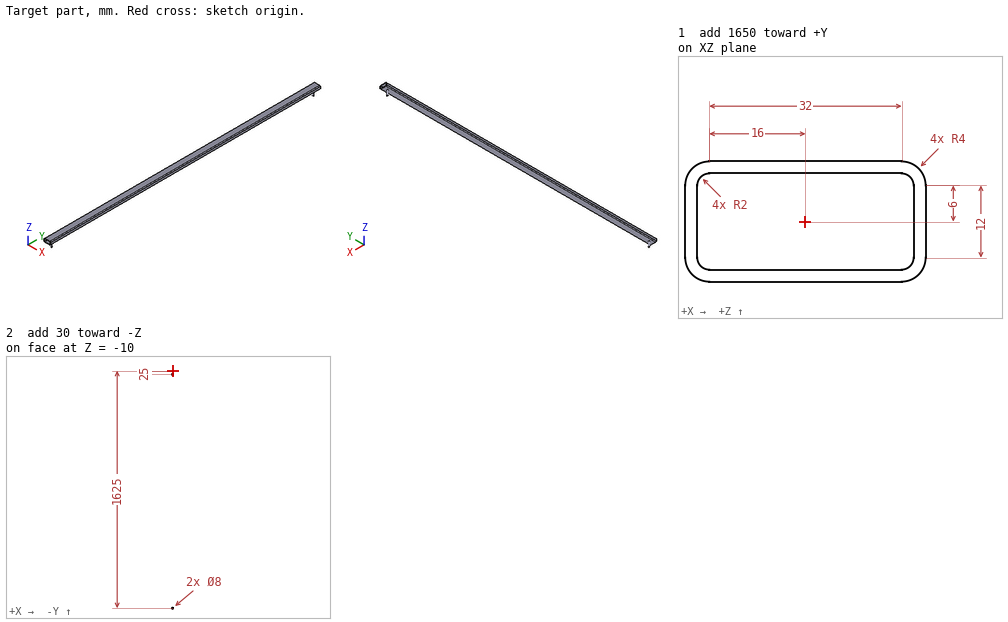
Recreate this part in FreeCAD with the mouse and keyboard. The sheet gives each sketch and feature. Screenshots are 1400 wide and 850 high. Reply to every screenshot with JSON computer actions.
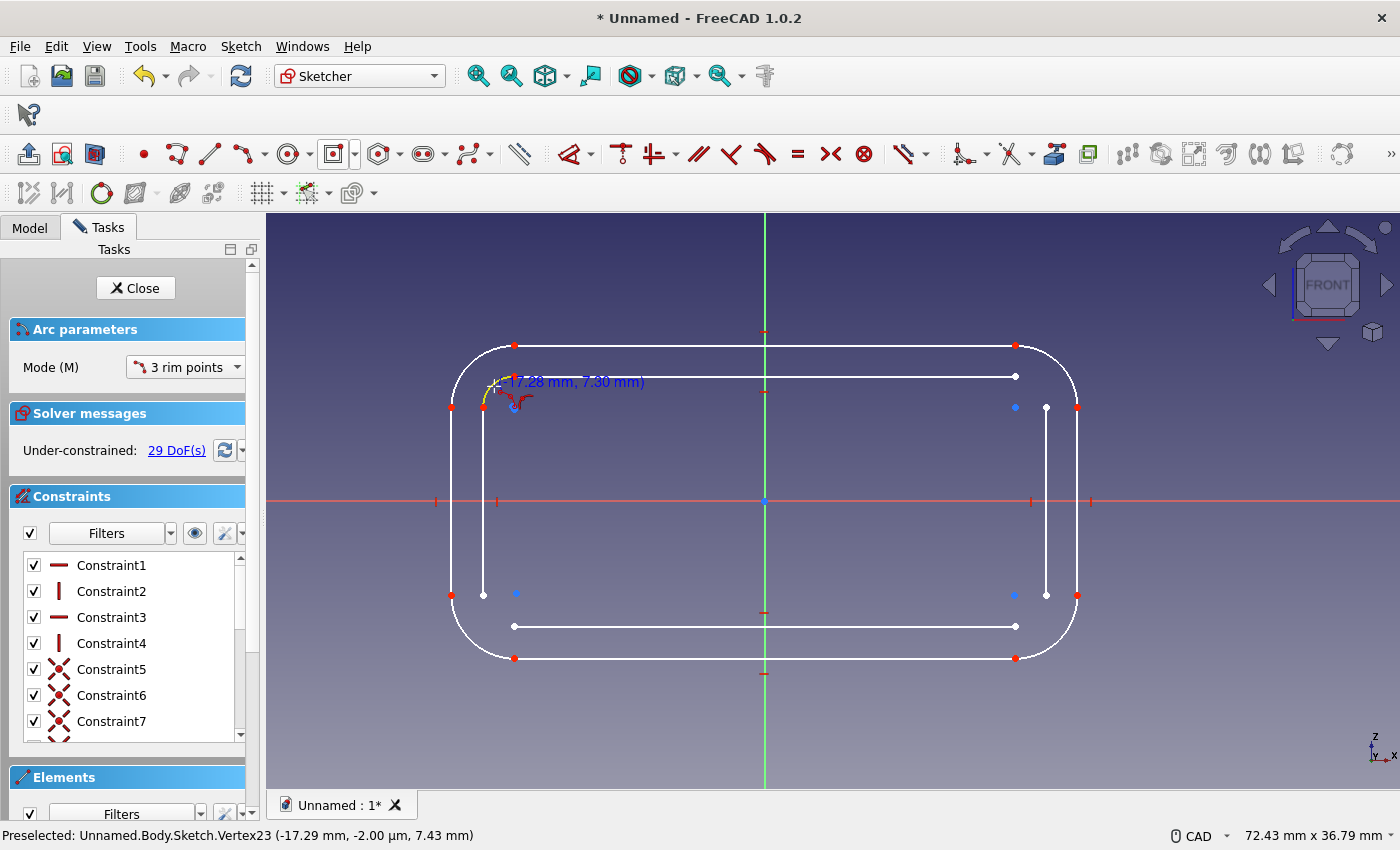
{"action": "left_click", "coordinate": [483, 596]}
{"action": "left_click", "coordinate": [514, 627]}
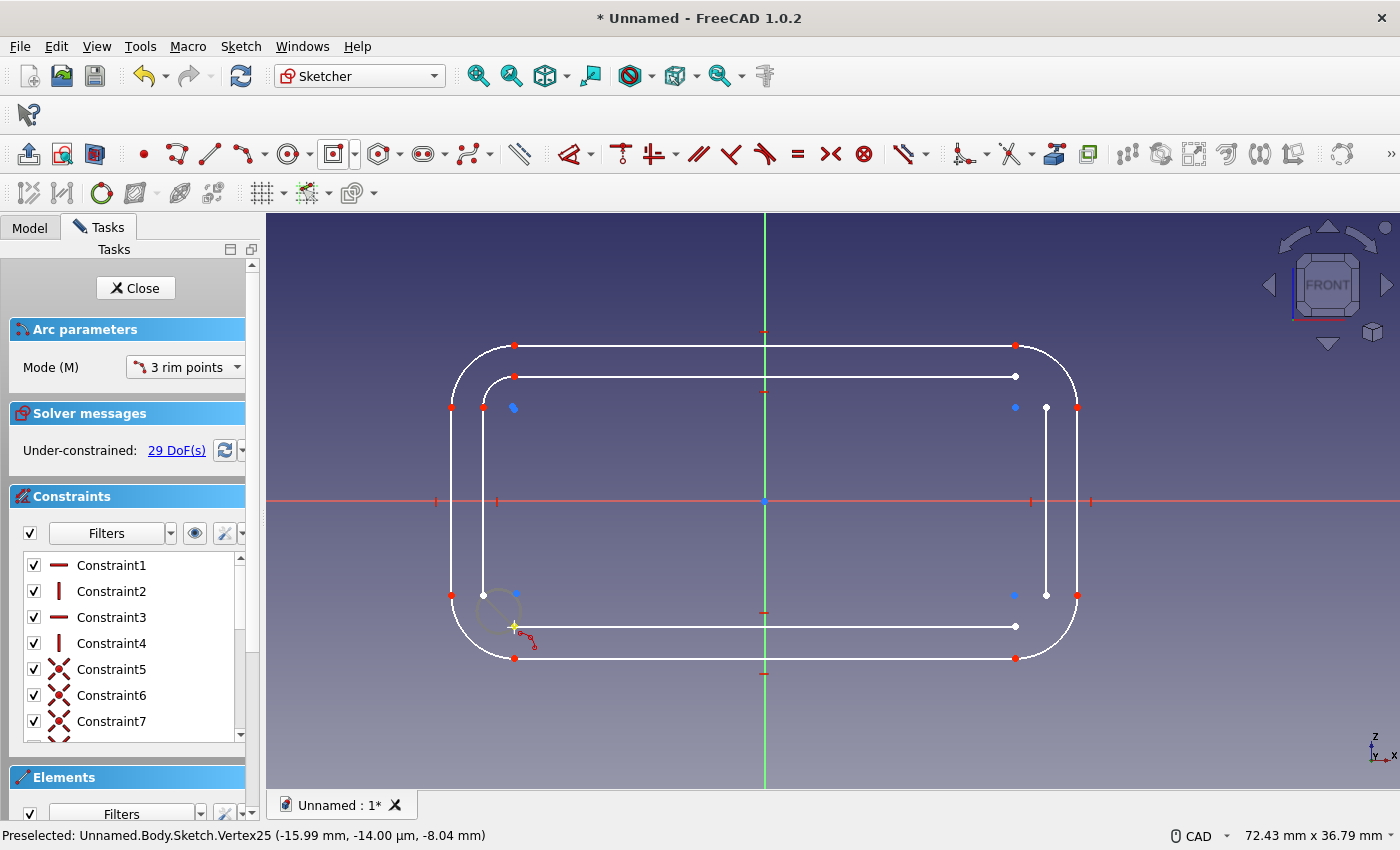
{"action": "scroll", "coordinate": [492, 617], "scroll_direction": "up", "scroll_amount": 3}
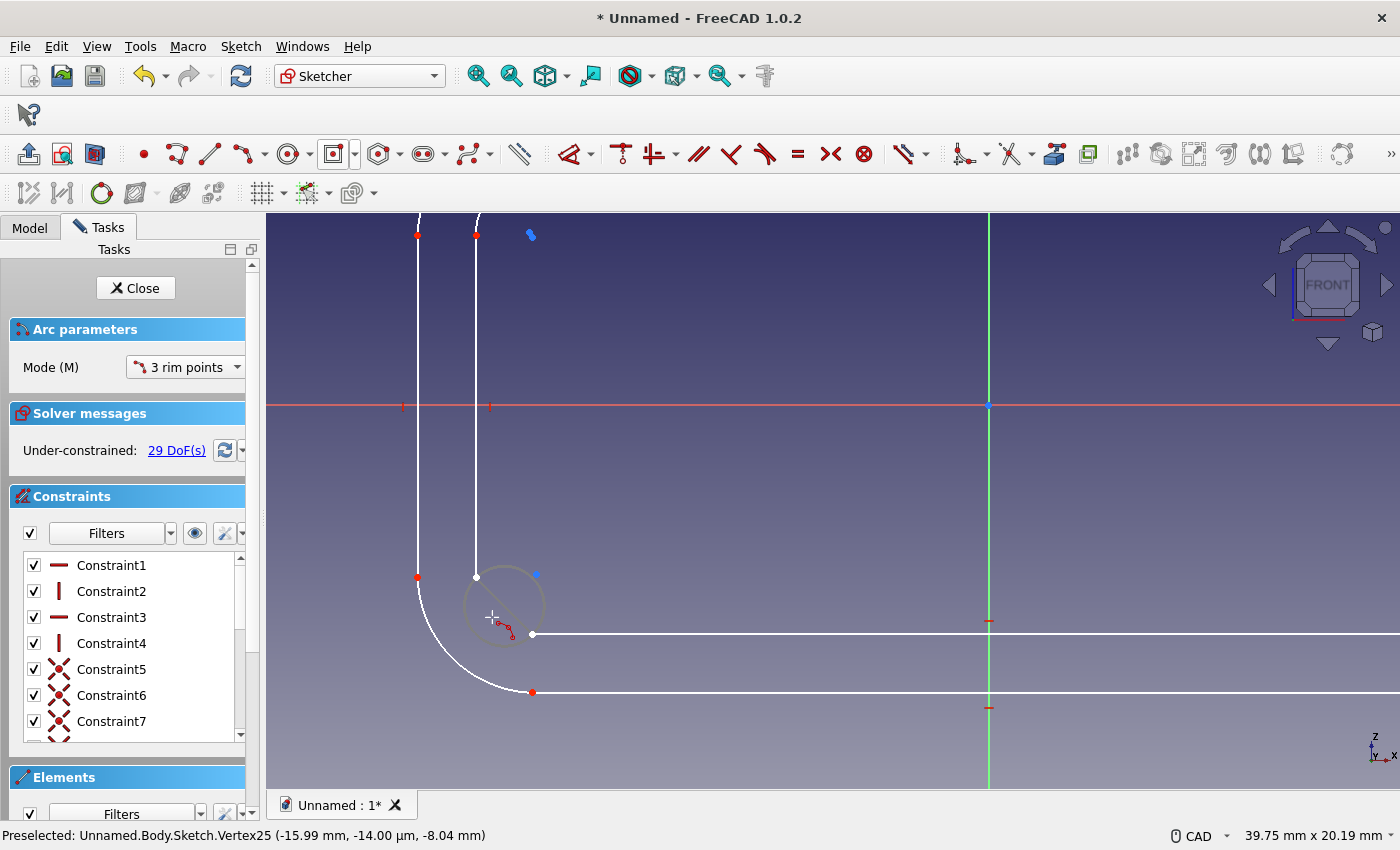
{"action": "left_click", "coordinate": [492, 617]}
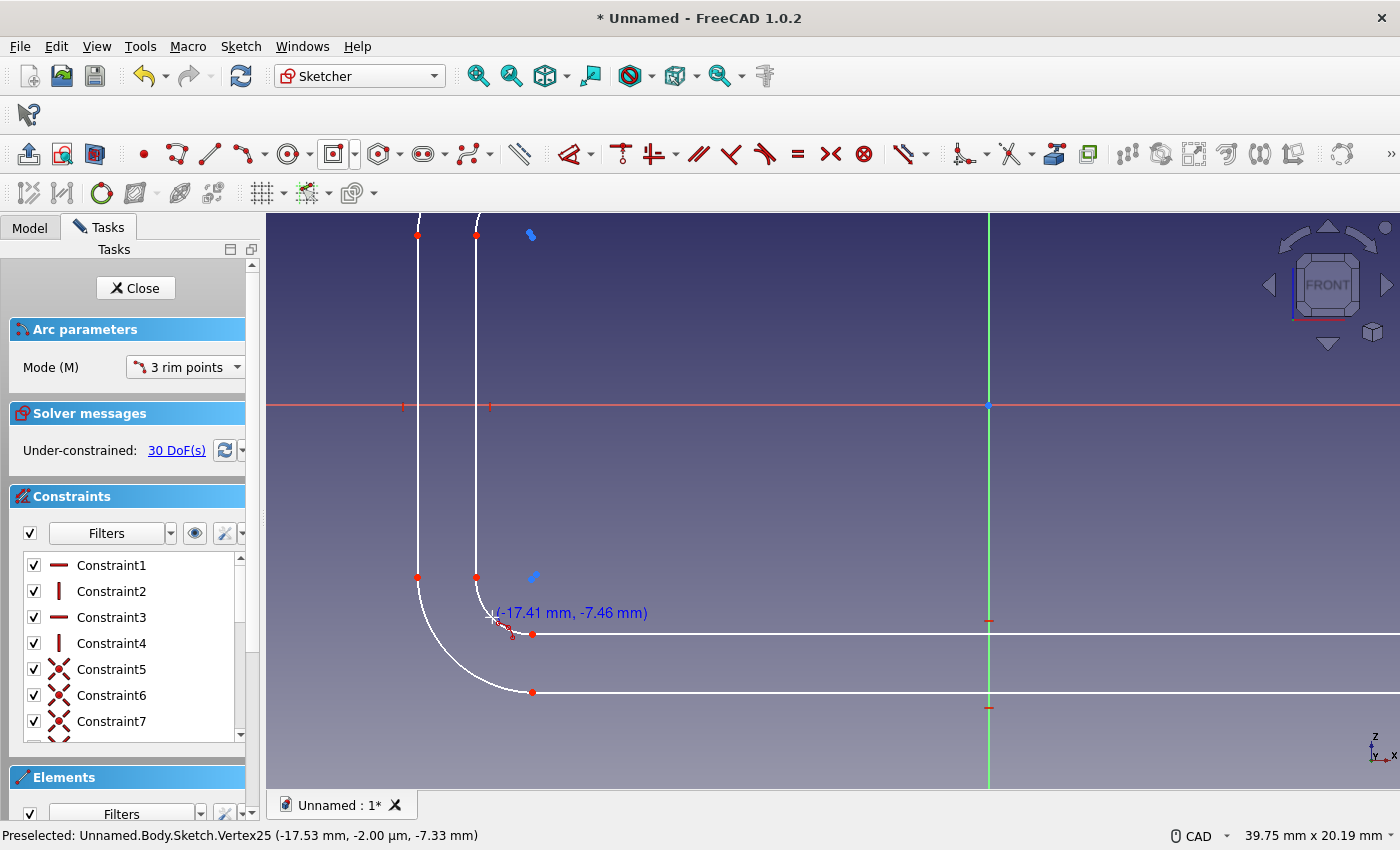
{"action": "scroll", "coordinate": [492, 618], "scroll_direction": "down", "scroll_amount": 3}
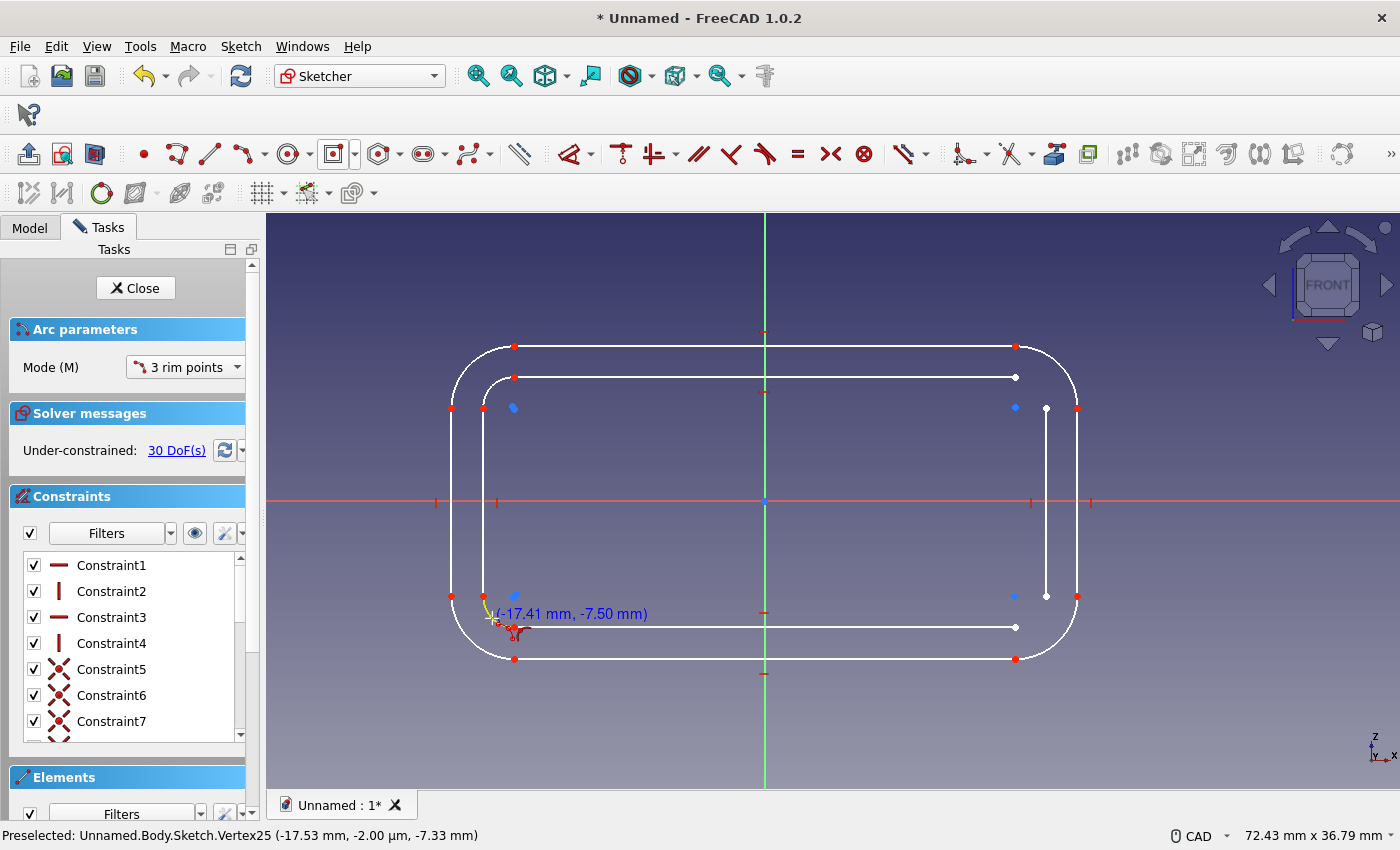
{"action": "left_click", "coordinate": [1015, 627]}
{"action": "left_click", "coordinate": [1046, 596]}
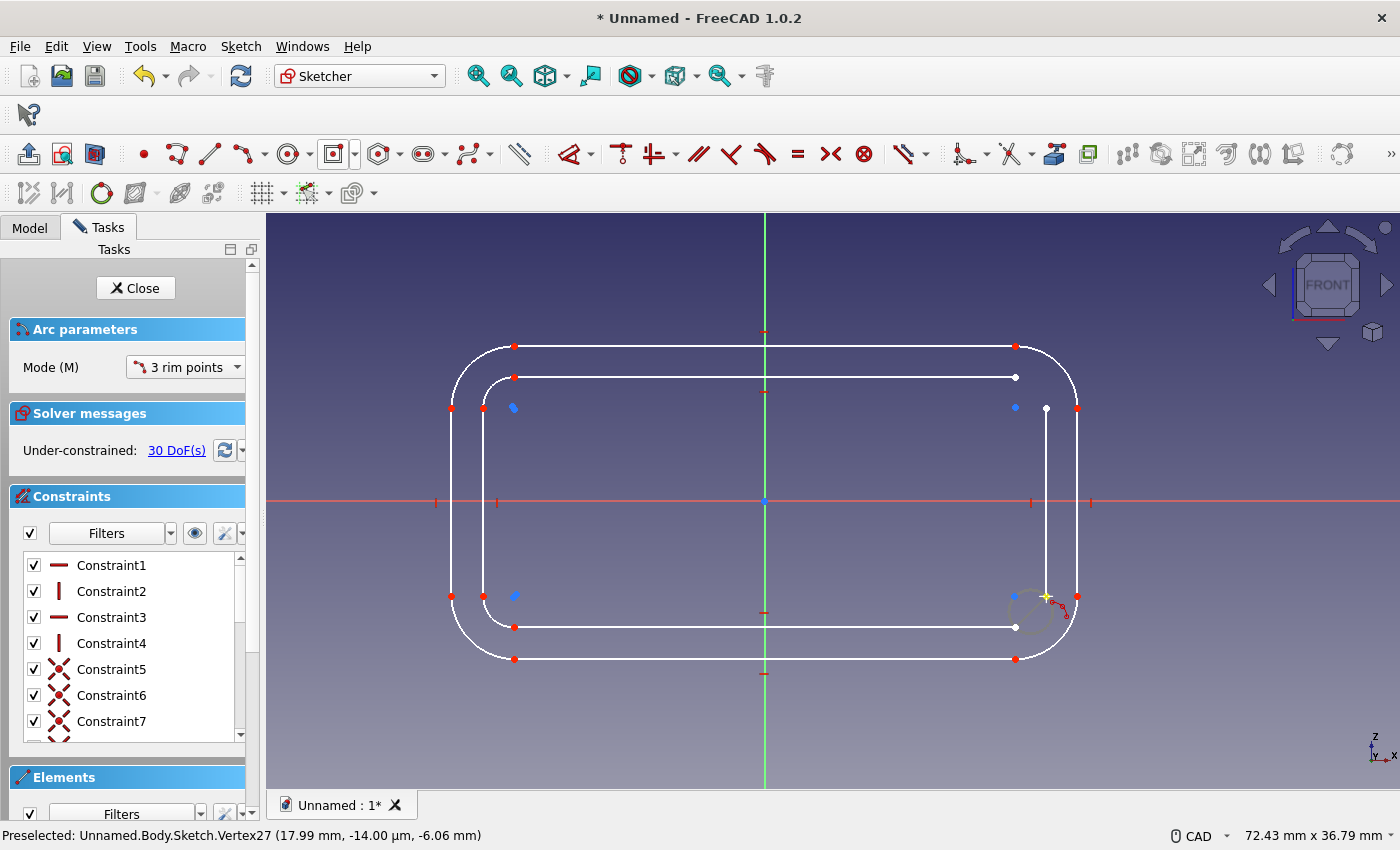
{"action": "scroll", "coordinate": [1037, 618], "scroll_direction": "up", "scroll_amount": 3}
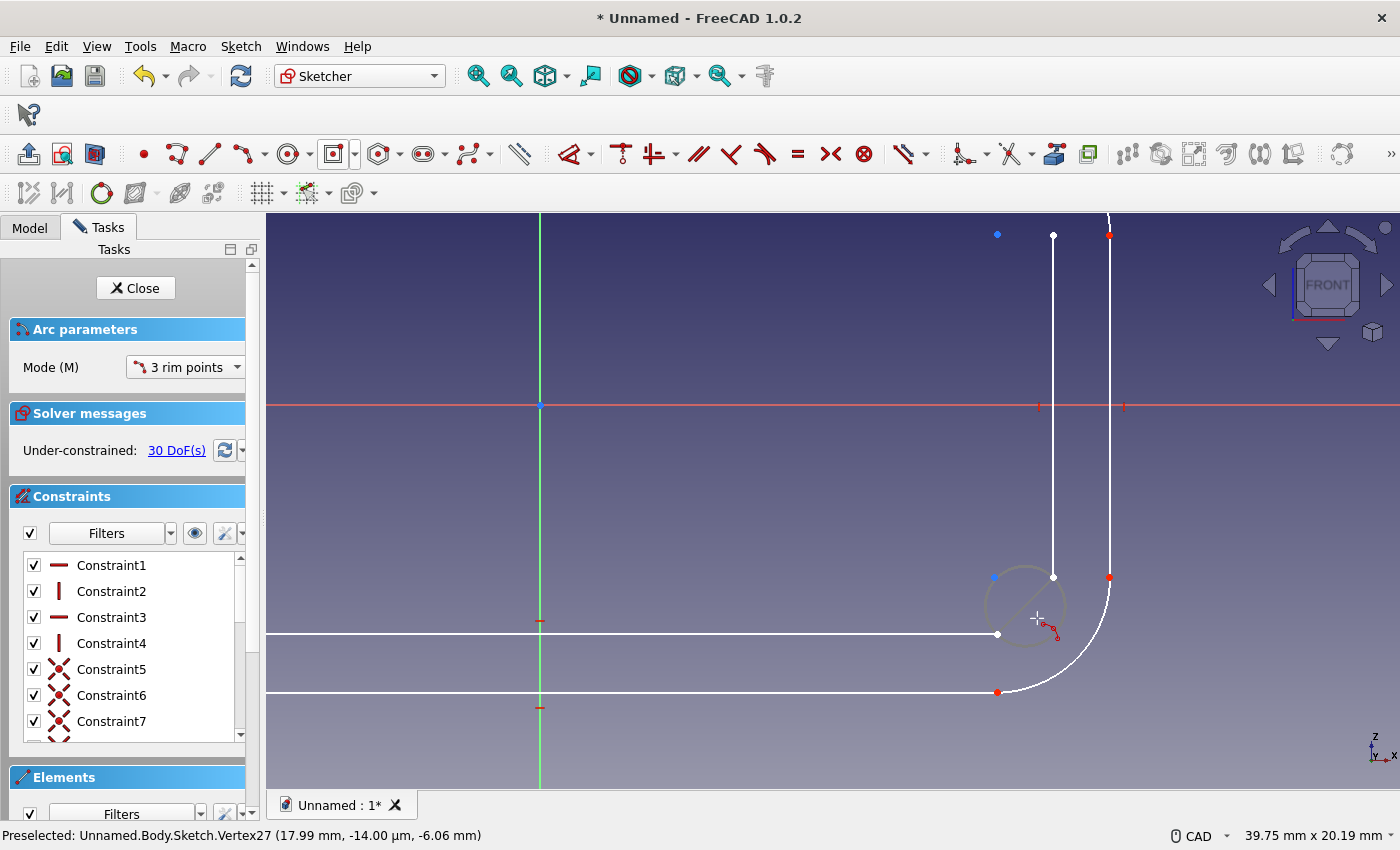
{"action": "left_click", "coordinate": [1037, 617]}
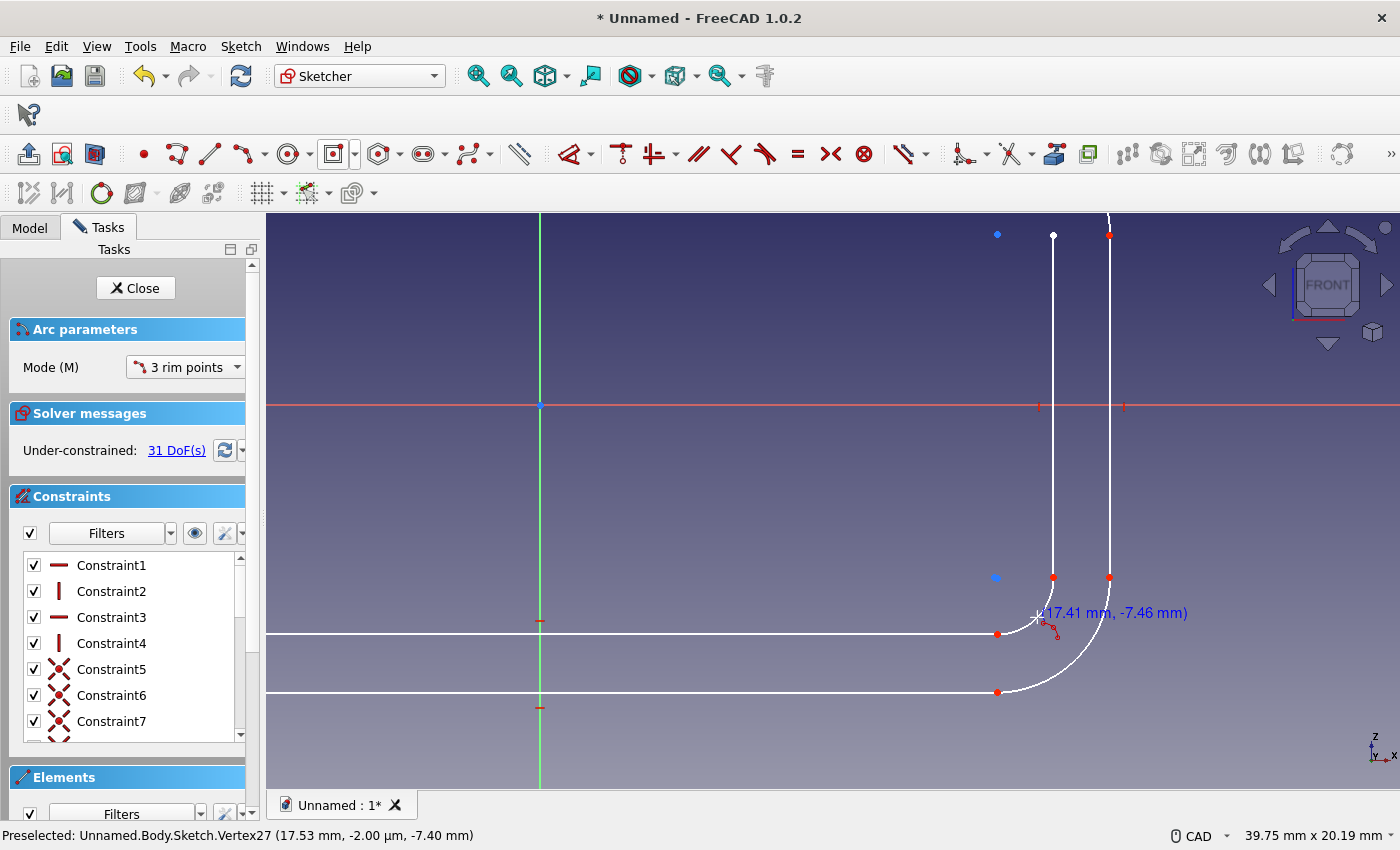
{"action": "scroll", "coordinate": [1037, 618], "scroll_direction": "down", "scroll_amount": 3}